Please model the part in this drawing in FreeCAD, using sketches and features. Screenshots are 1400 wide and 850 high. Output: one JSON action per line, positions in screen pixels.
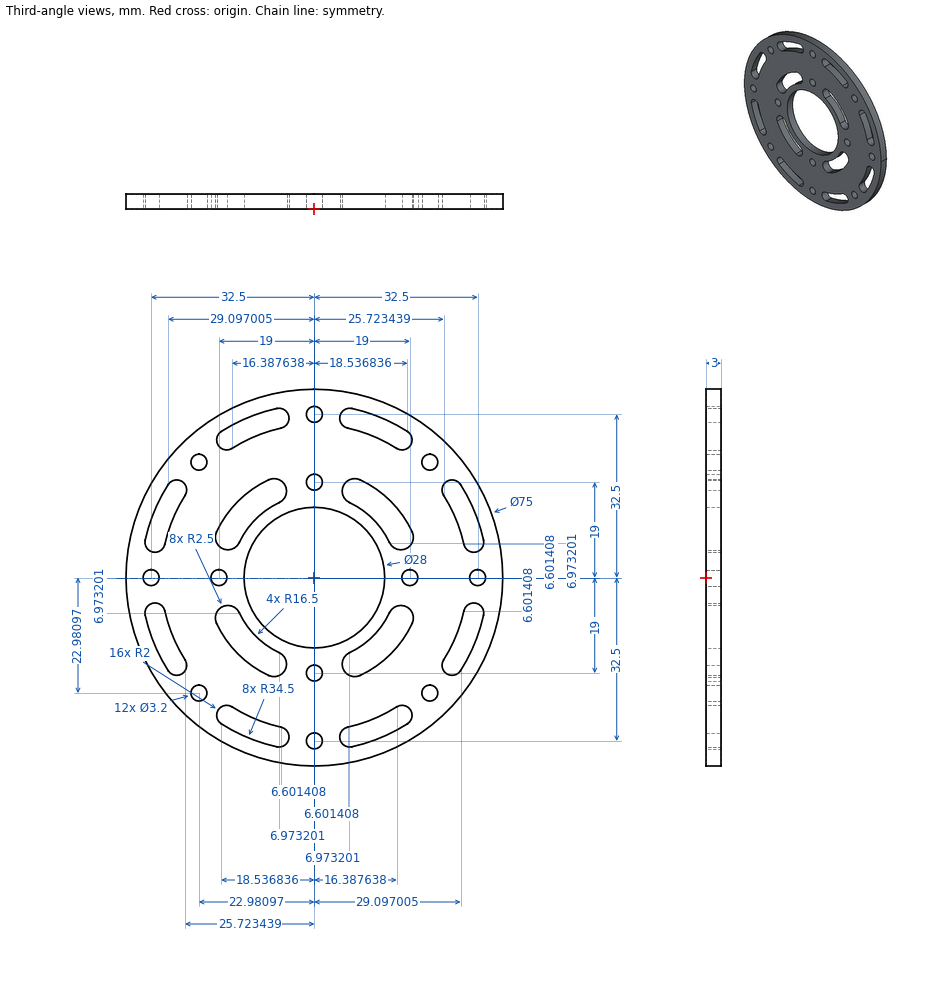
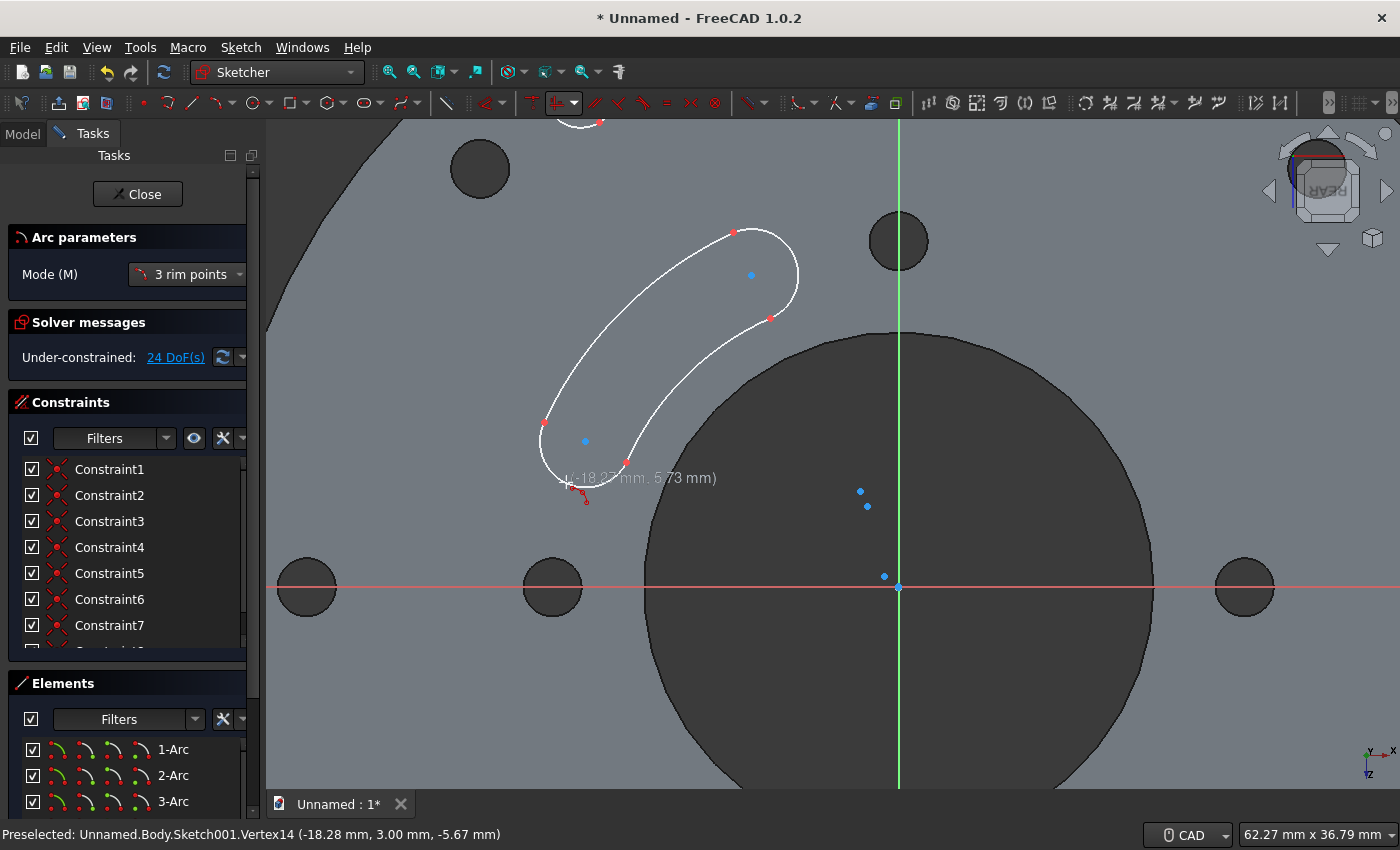
{"action": "scroll", "coordinate": [686, 376], "scroll_direction": "down", "scroll_amount": 5}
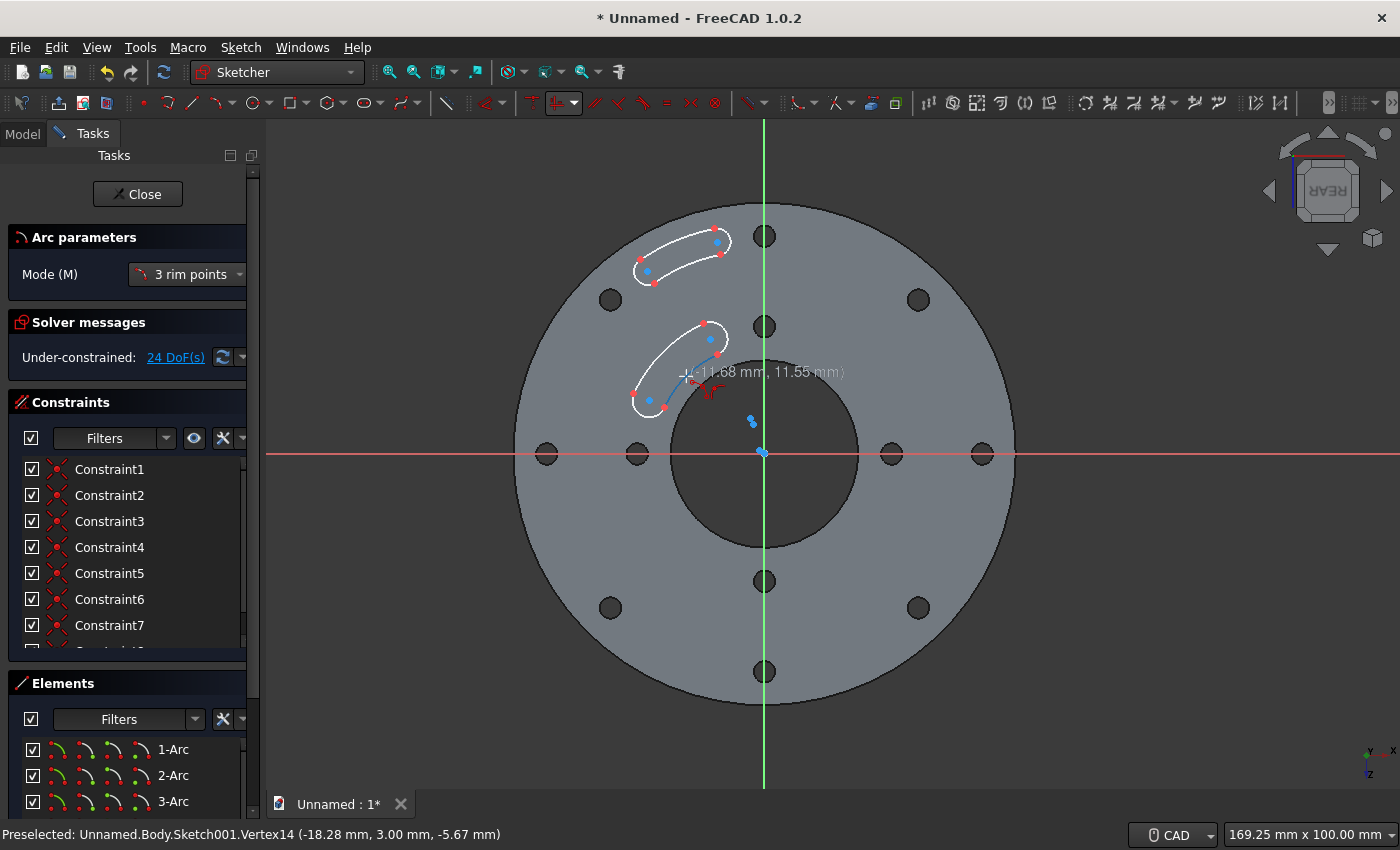
{"action": "left_click", "coordinate": [809, 254]}
{"action": "left_click", "coordinate": [874, 282]}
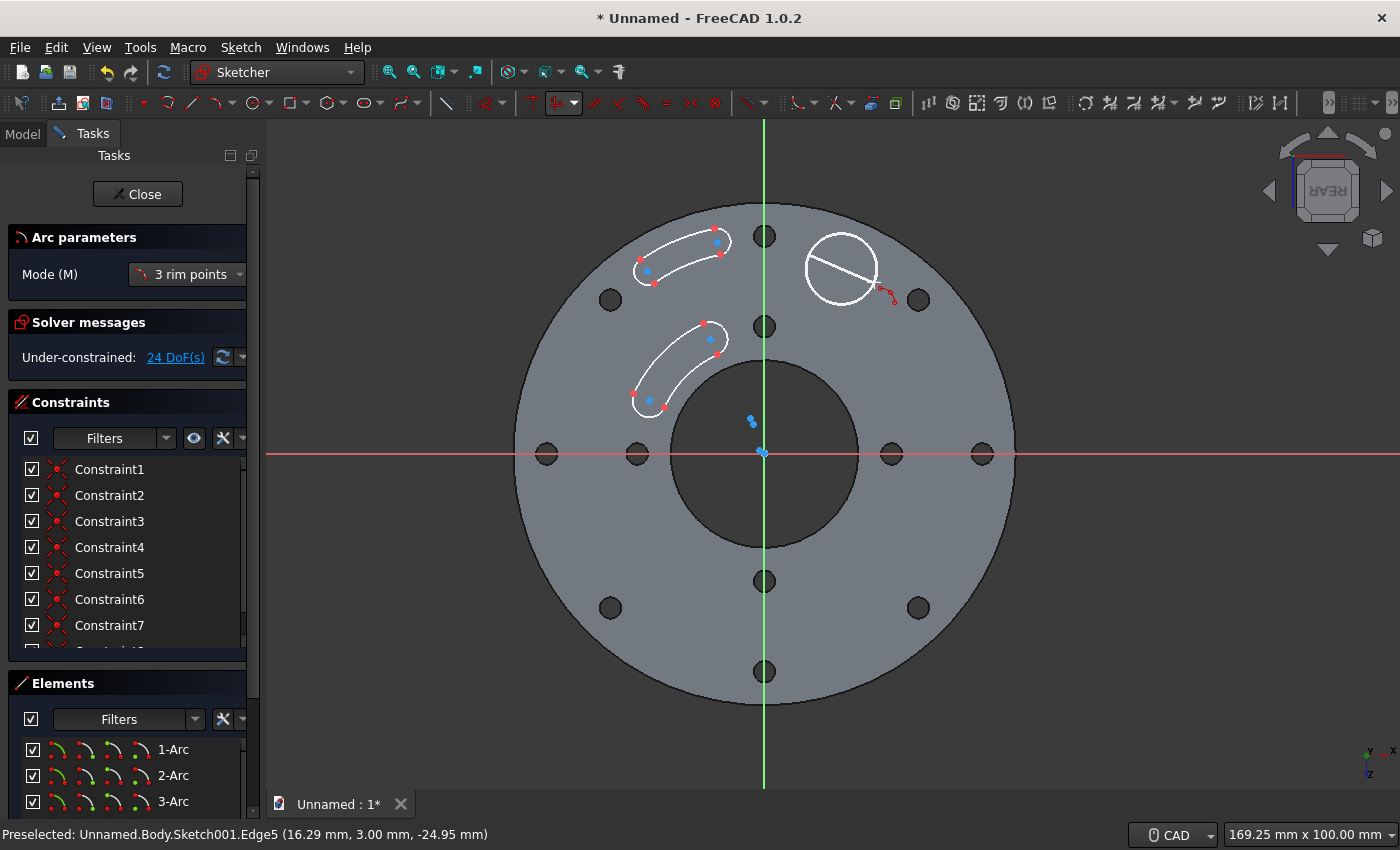
{"action": "scroll", "coordinate": [843, 265], "scroll_direction": "up", "scroll_amount": 9}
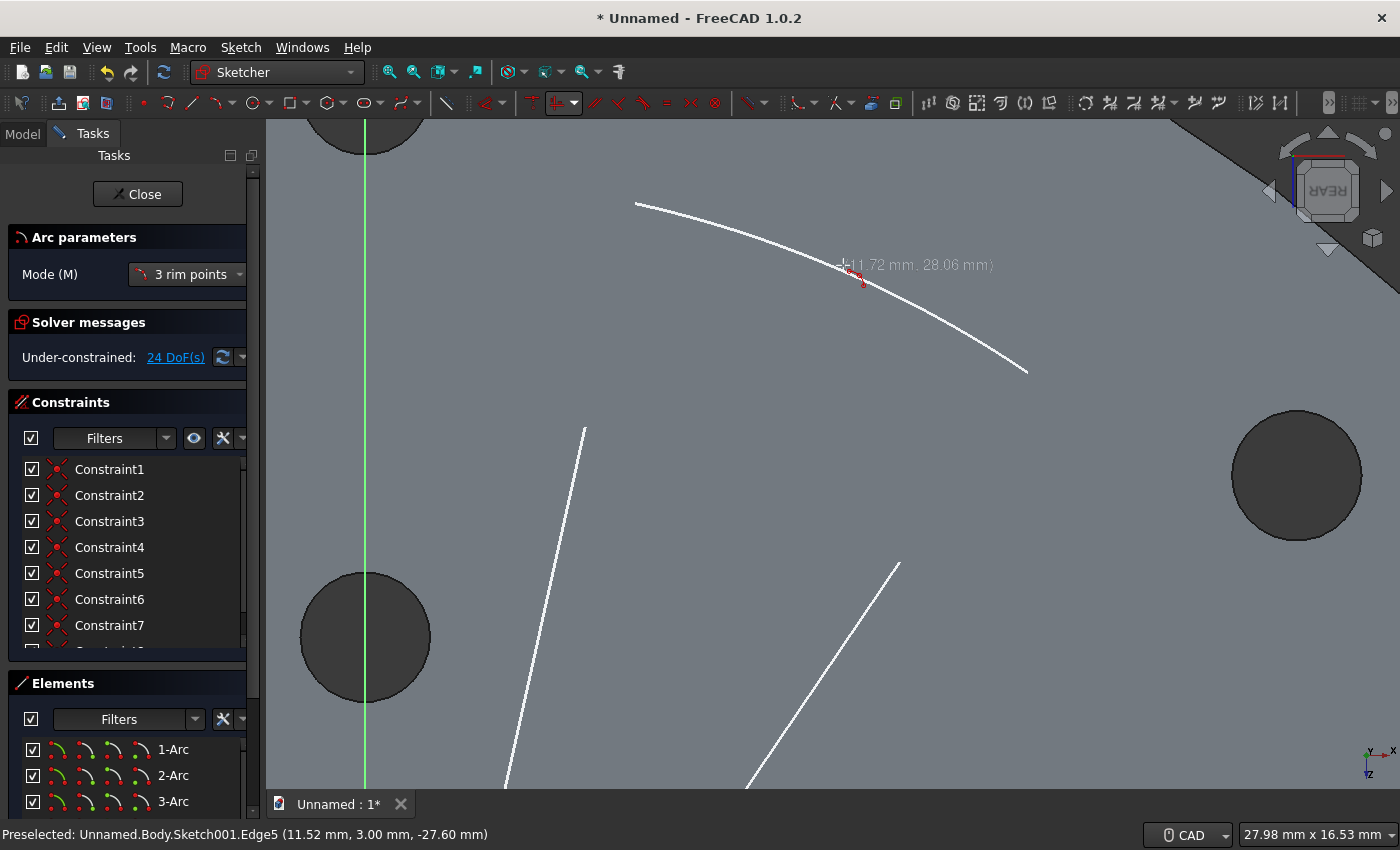
{"action": "left_click", "coordinate": [838, 265]}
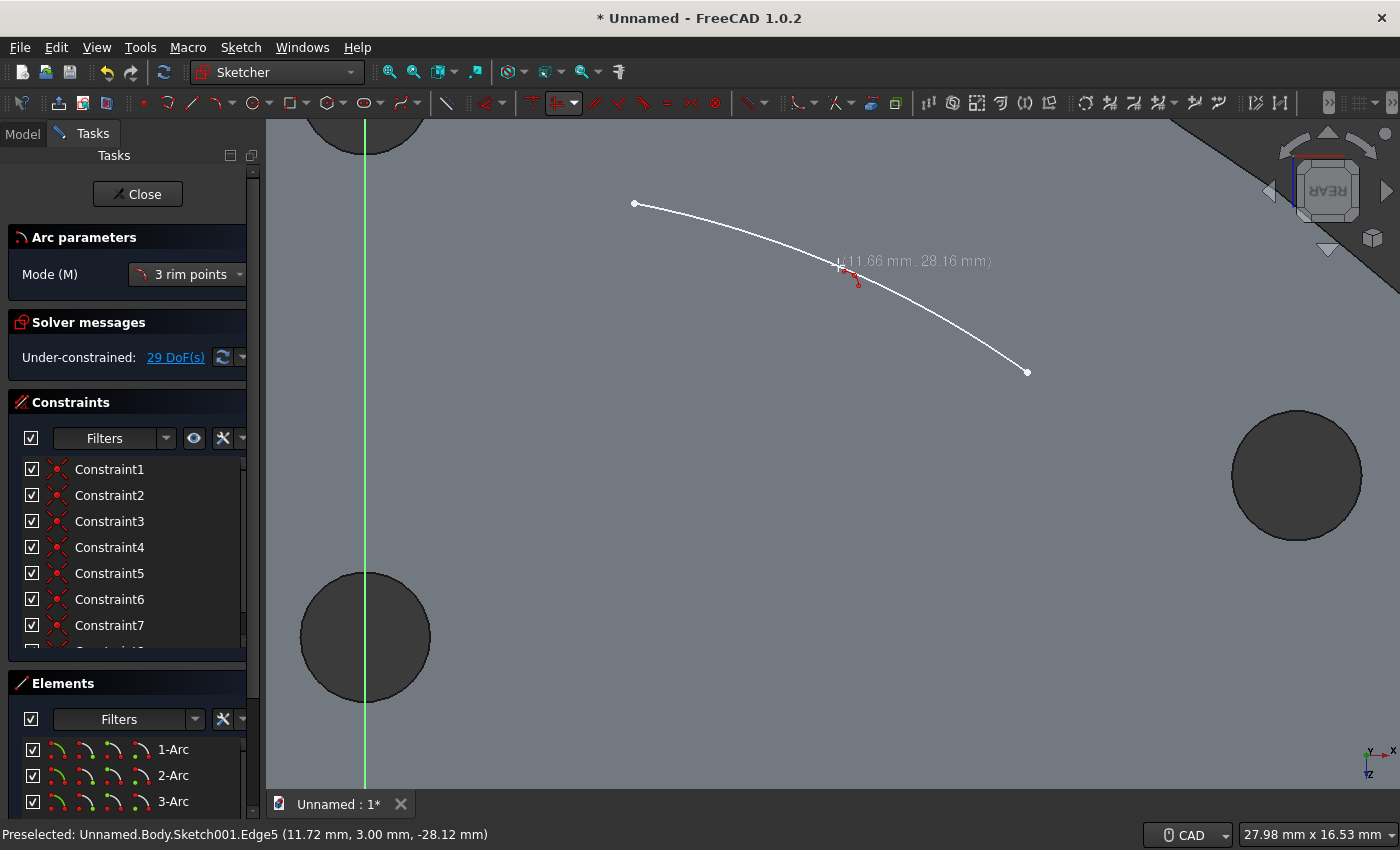
{"action": "scroll", "coordinate": [844, 265], "scroll_direction": "down", "scroll_amount": 9}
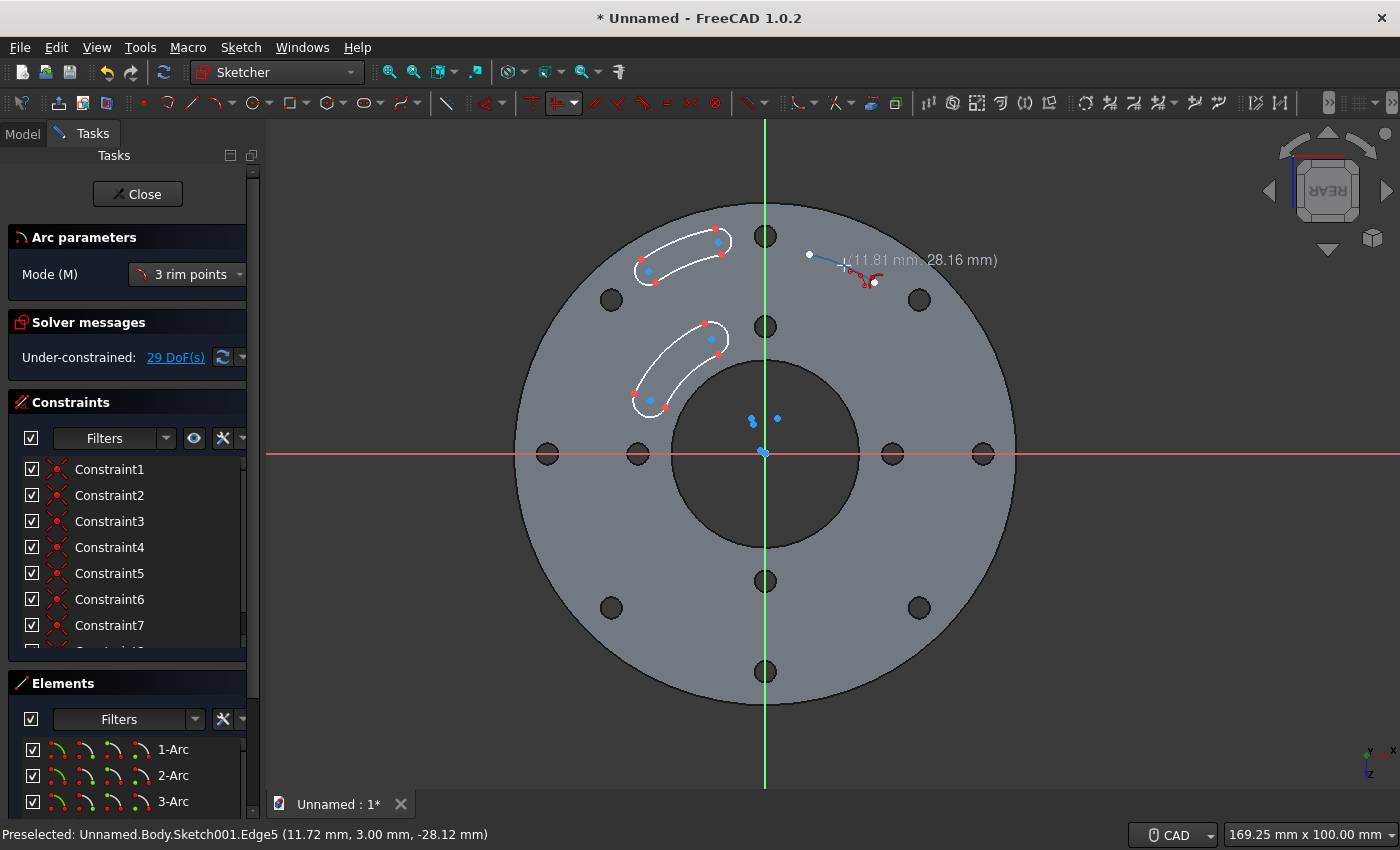
{"action": "left_click", "coordinate": [875, 283]}
{"action": "left_click", "coordinate": [890, 259]}
{"action": "left_click", "coordinate": [894, 278]}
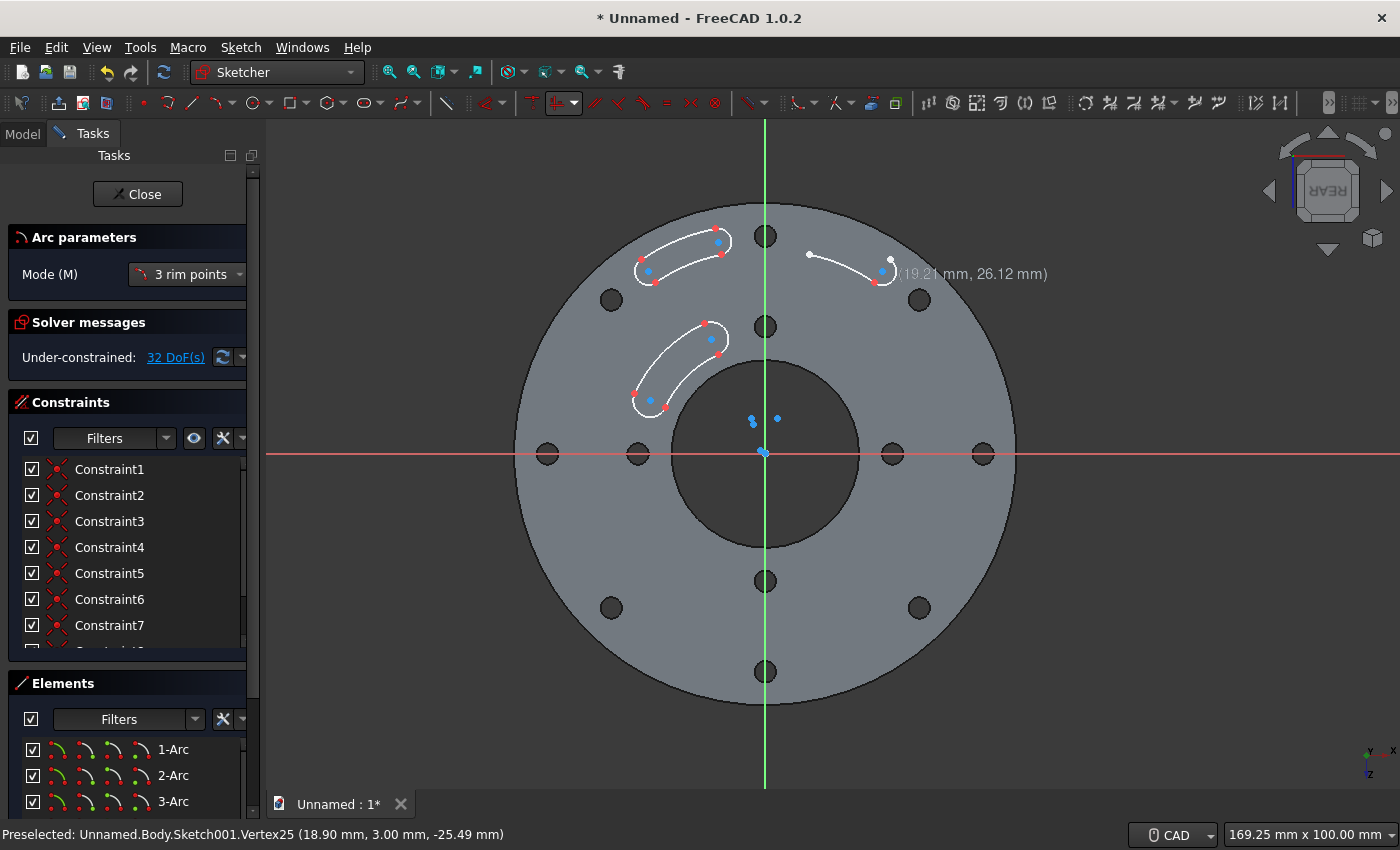
{"action": "left_click", "coordinate": [890, 260]}
{"action": "left_click", "coordinate": [815, 228]}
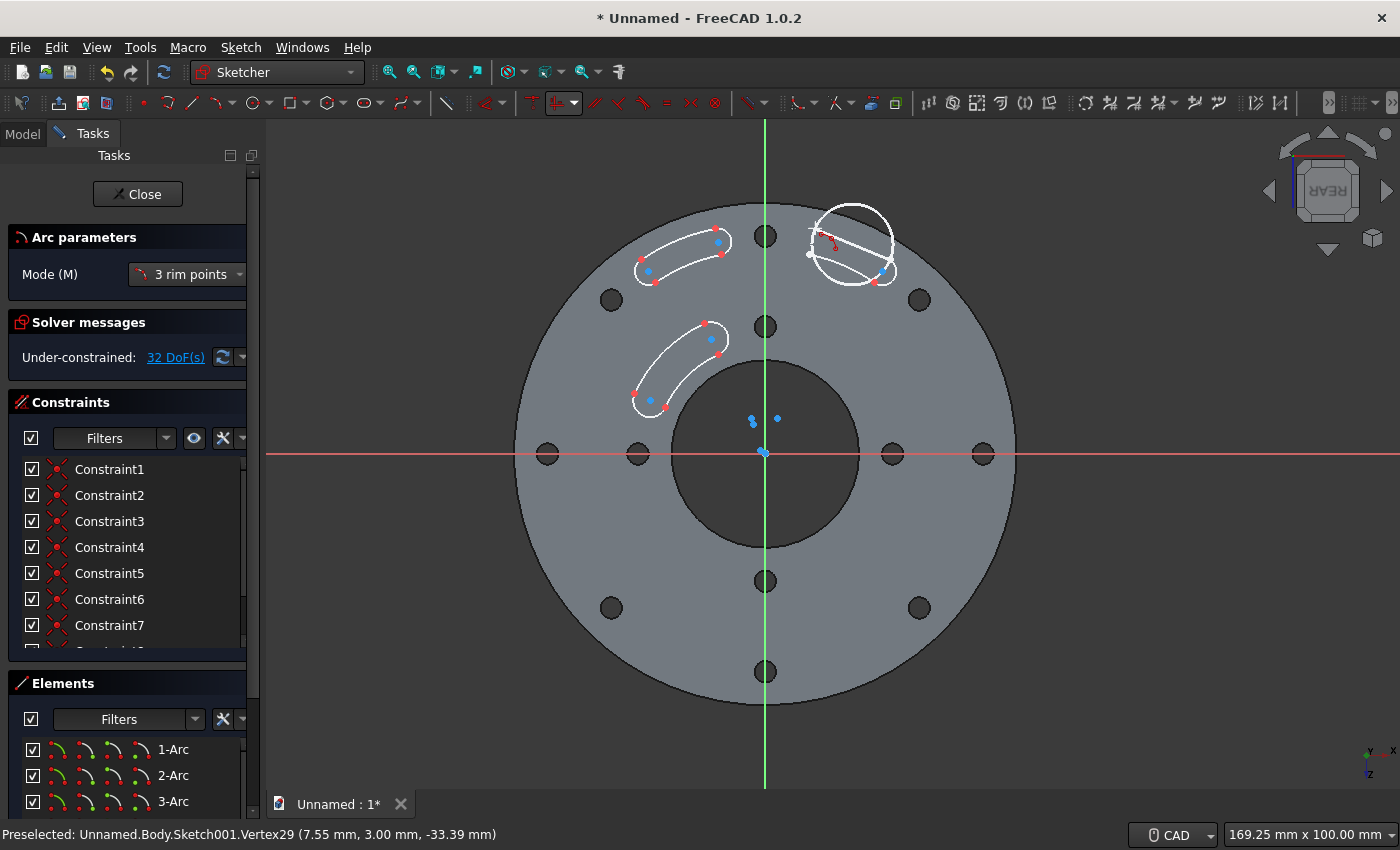
{"action": "scroll", "coordinate": [854, 240], "scroll_direction": "up", "scroll_amount": 8}